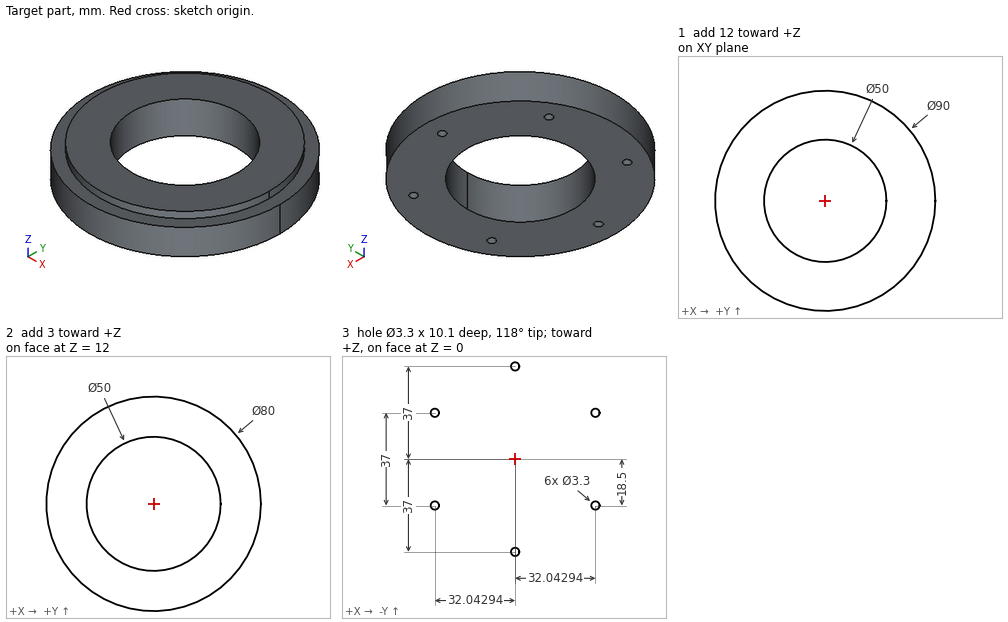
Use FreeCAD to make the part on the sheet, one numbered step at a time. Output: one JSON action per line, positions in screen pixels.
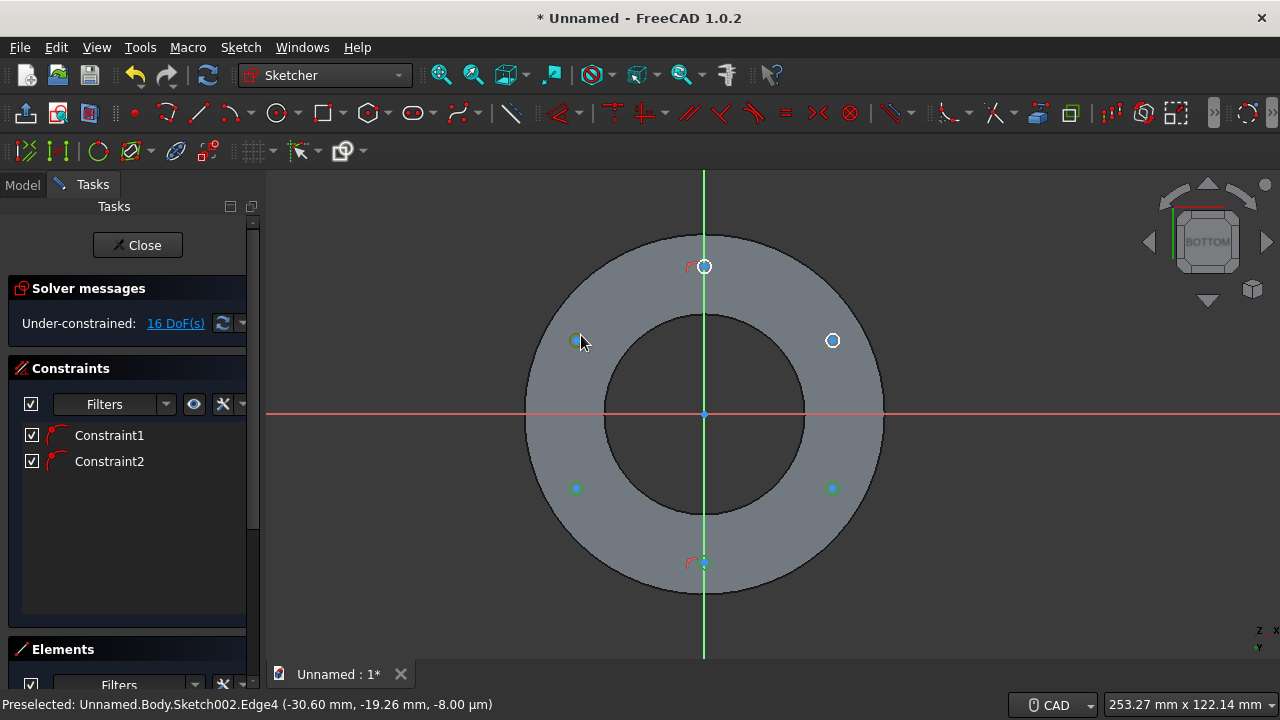
{"action": "scroll", "coordinate": [709, 262], "scroll_direction": "up", "scroll_amount": 6}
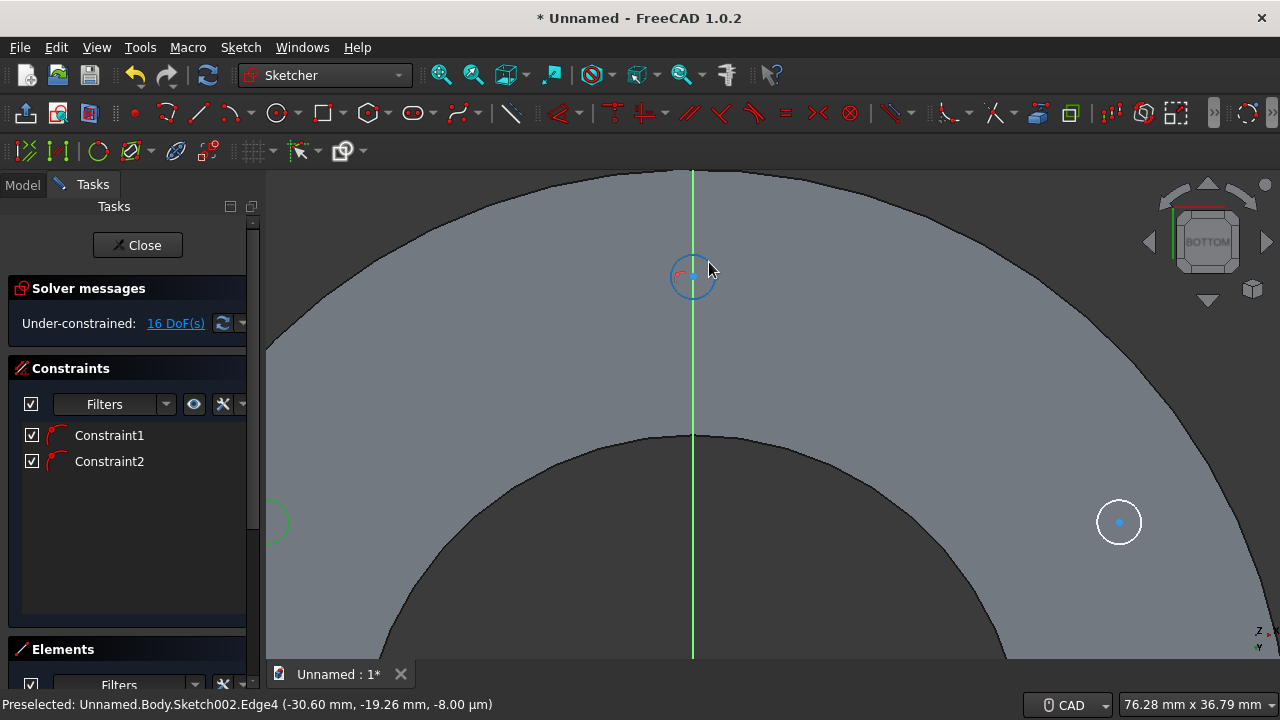
{"action": "left_click", "coordinate": [709, 261]}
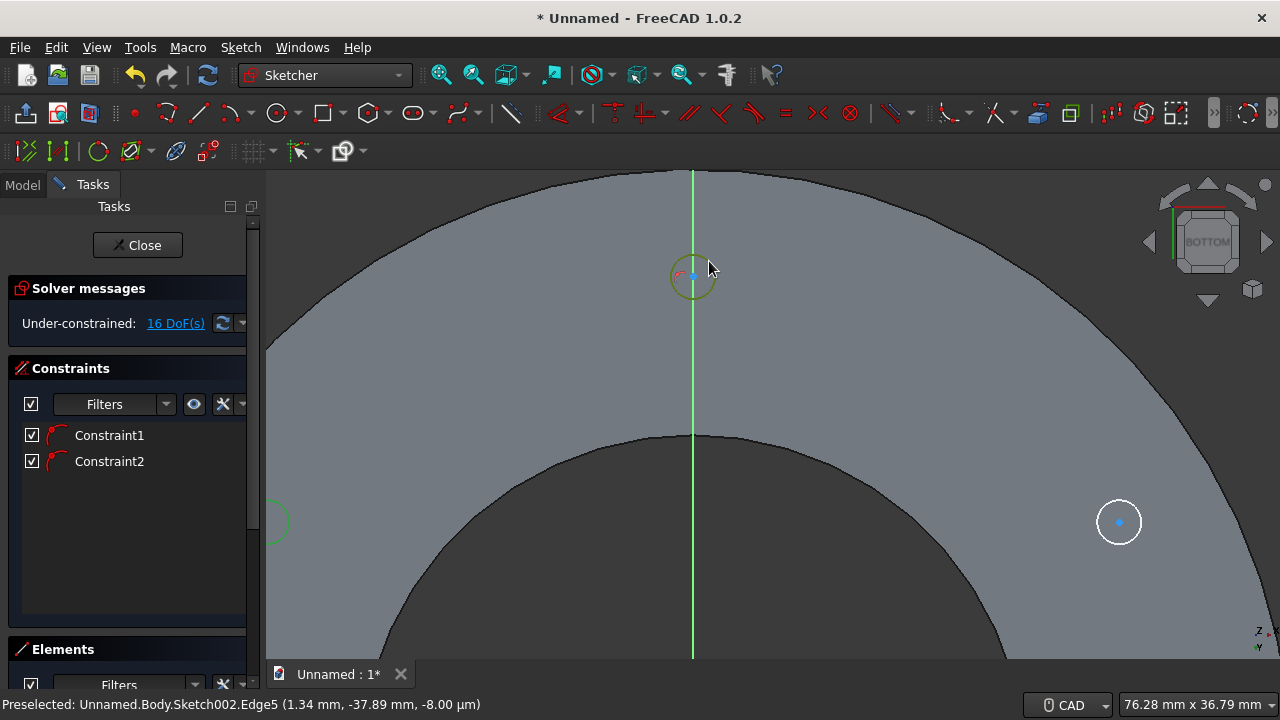
{"action": "left_click", "coordinate": [1104, 507]}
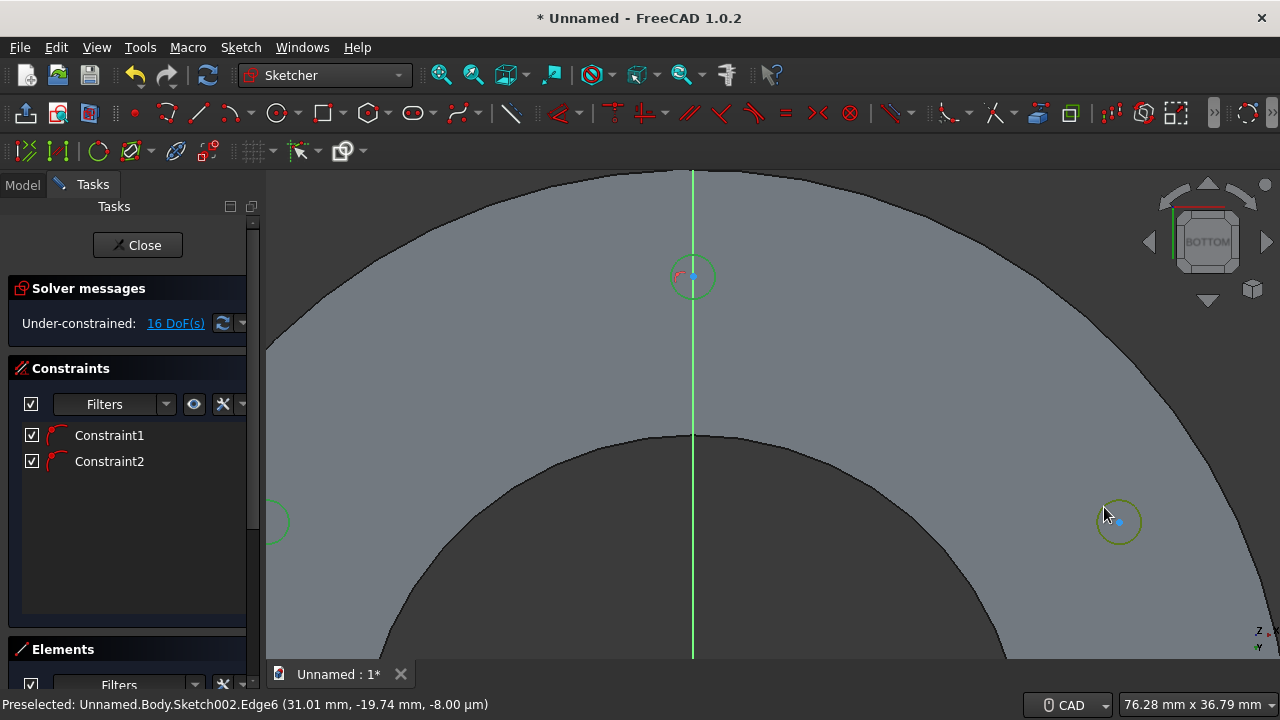
{"action": "left_click", "coordinate": [786, 114]}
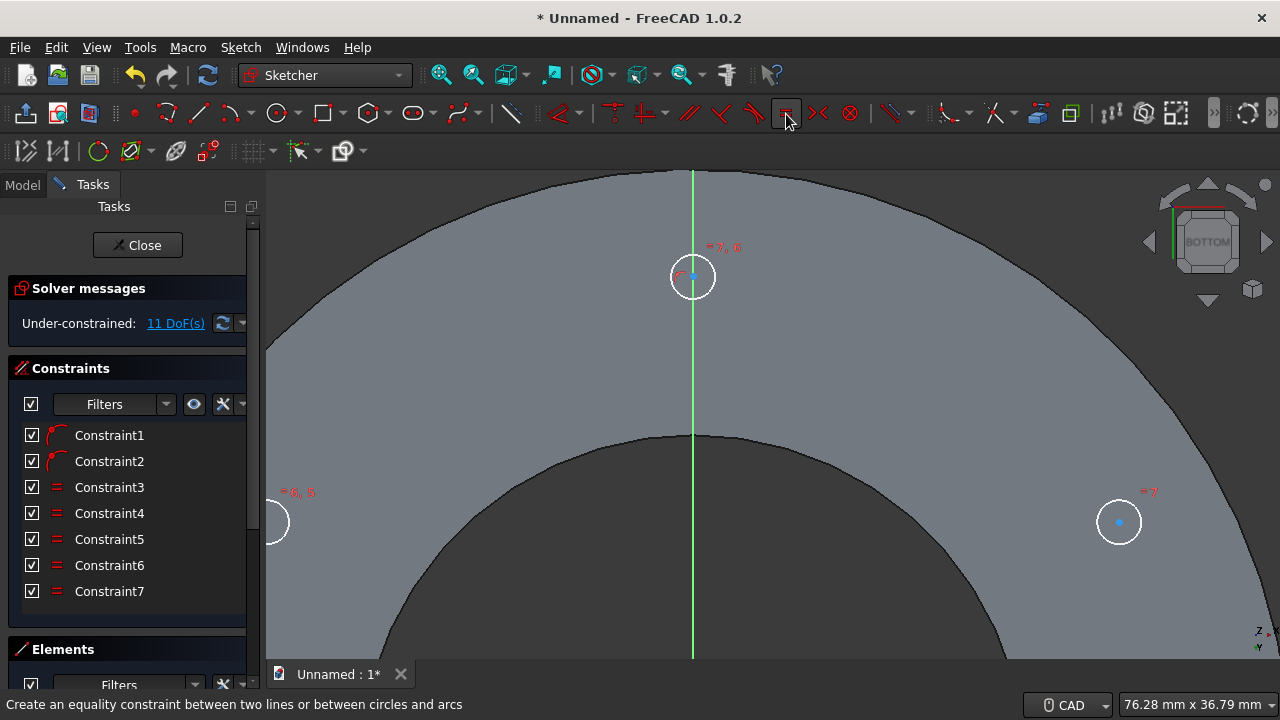
{"action": "scroll", "coordinate": [709, 262], "scroll_direction": "down", "scroll_amount": 6}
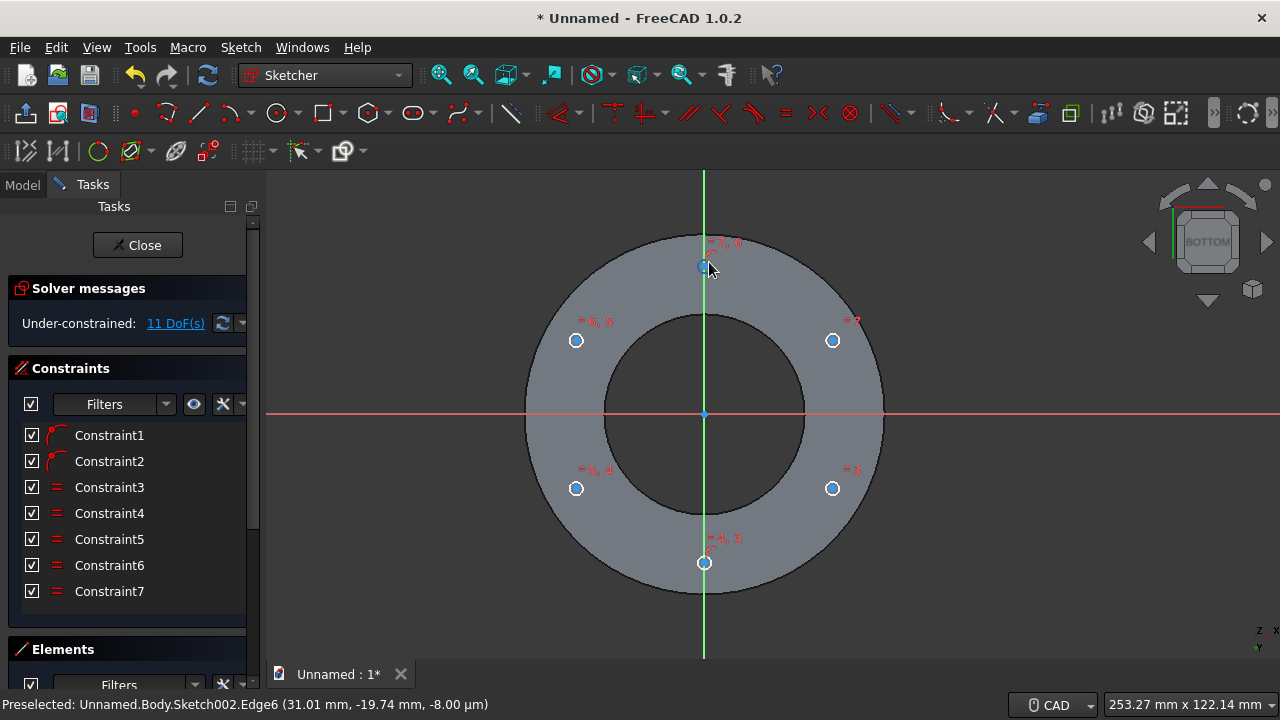
{"action": "left_click", "coordinate": [833, 489]}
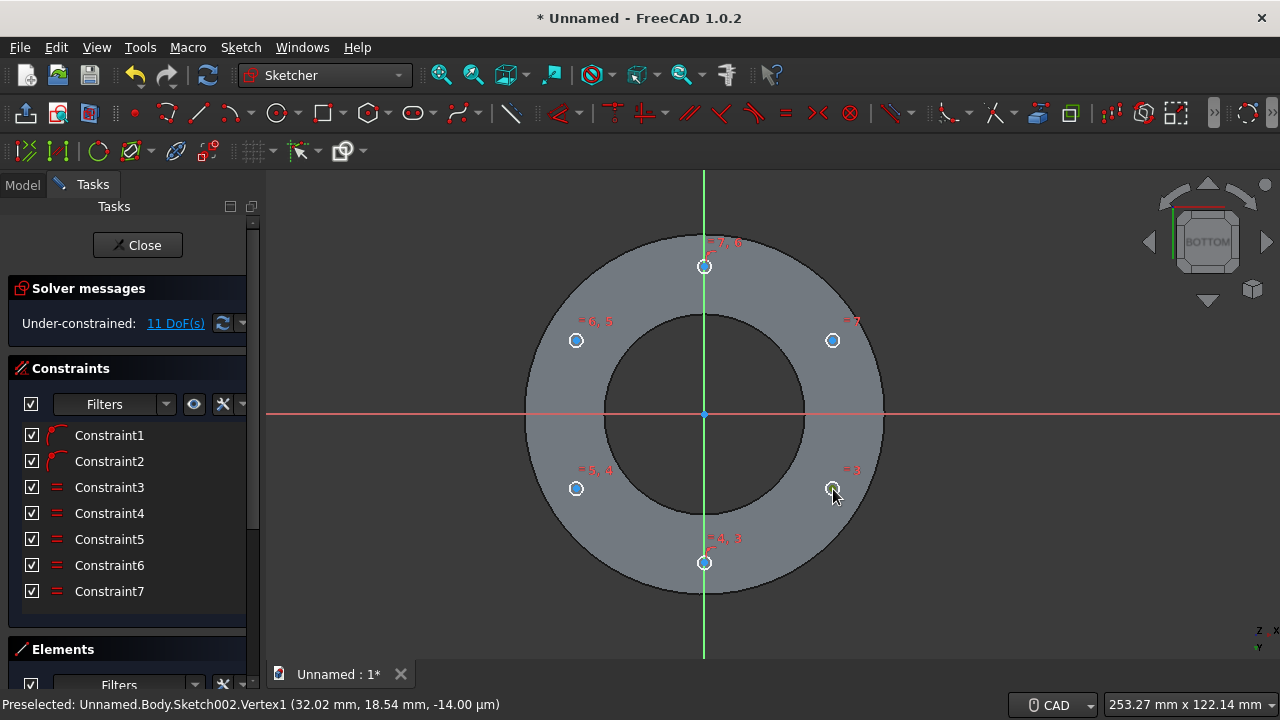
{"action": "left_click", "coordinate": [576, 489]}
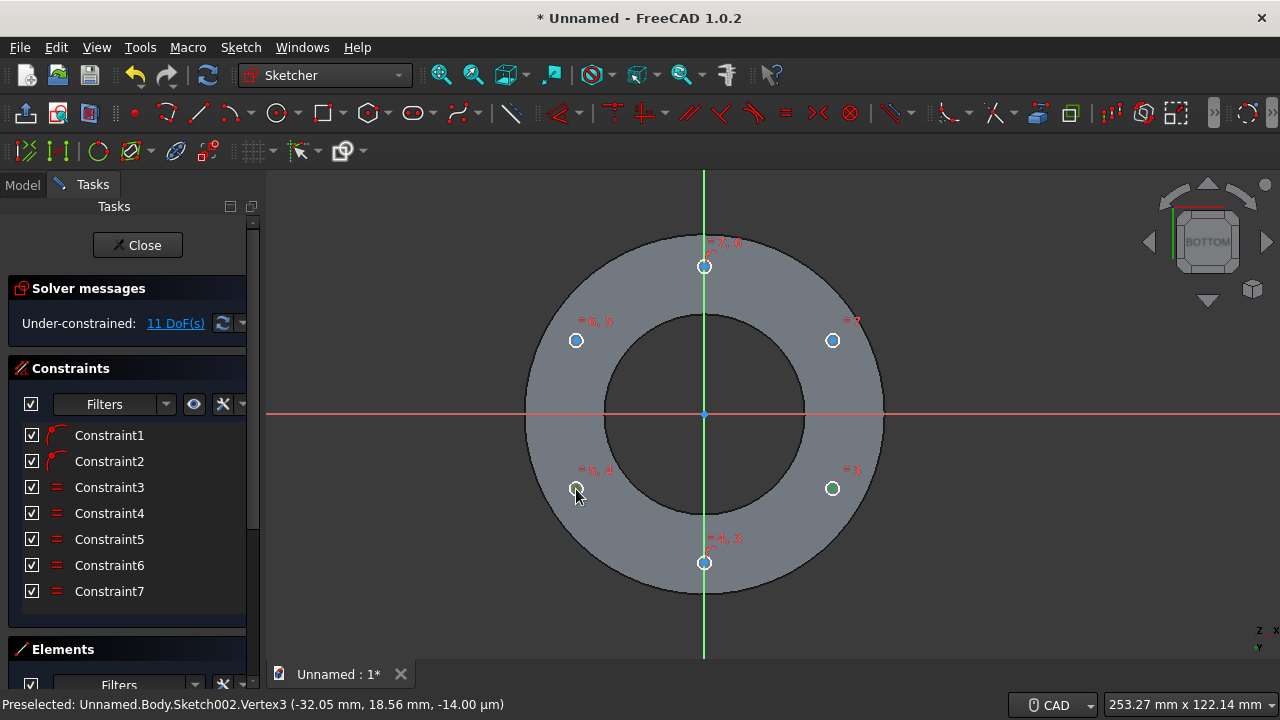
{"action": "left_click", "coordinate": [668, 114]}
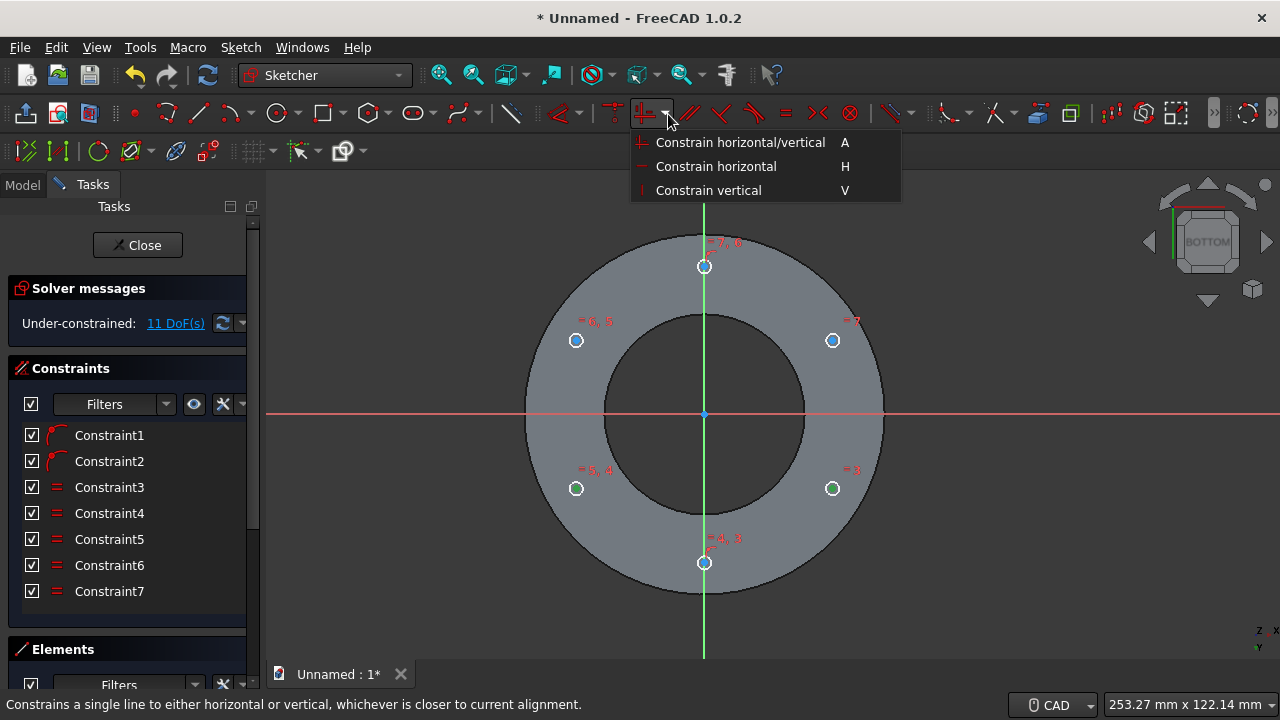
{"action": "left_click", "coordinate": [766, 166]}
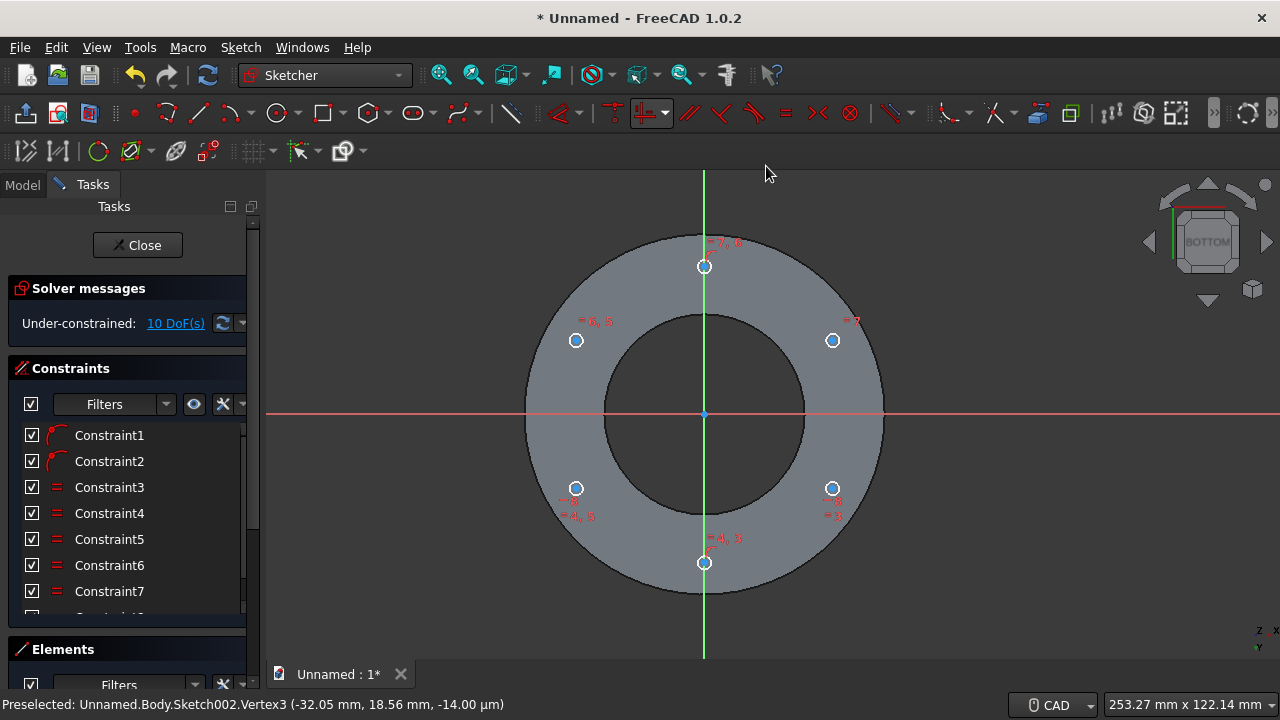
{"action": "left_click", "coordinate": [576, 489]}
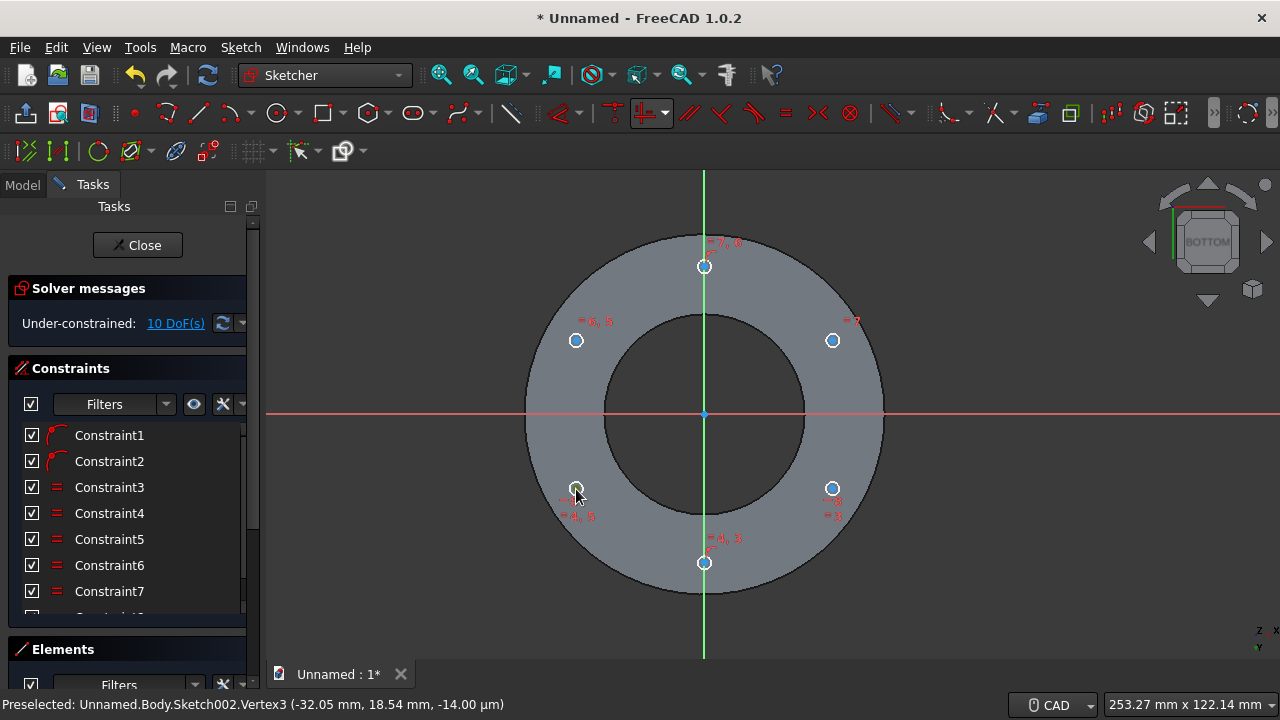
{"action": "left_click", "coordinate": [576, 341]}